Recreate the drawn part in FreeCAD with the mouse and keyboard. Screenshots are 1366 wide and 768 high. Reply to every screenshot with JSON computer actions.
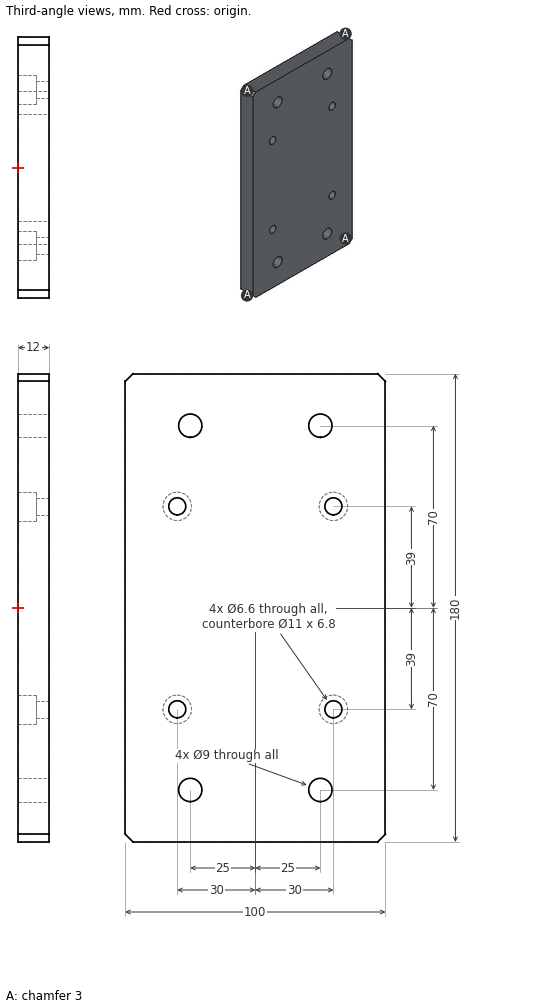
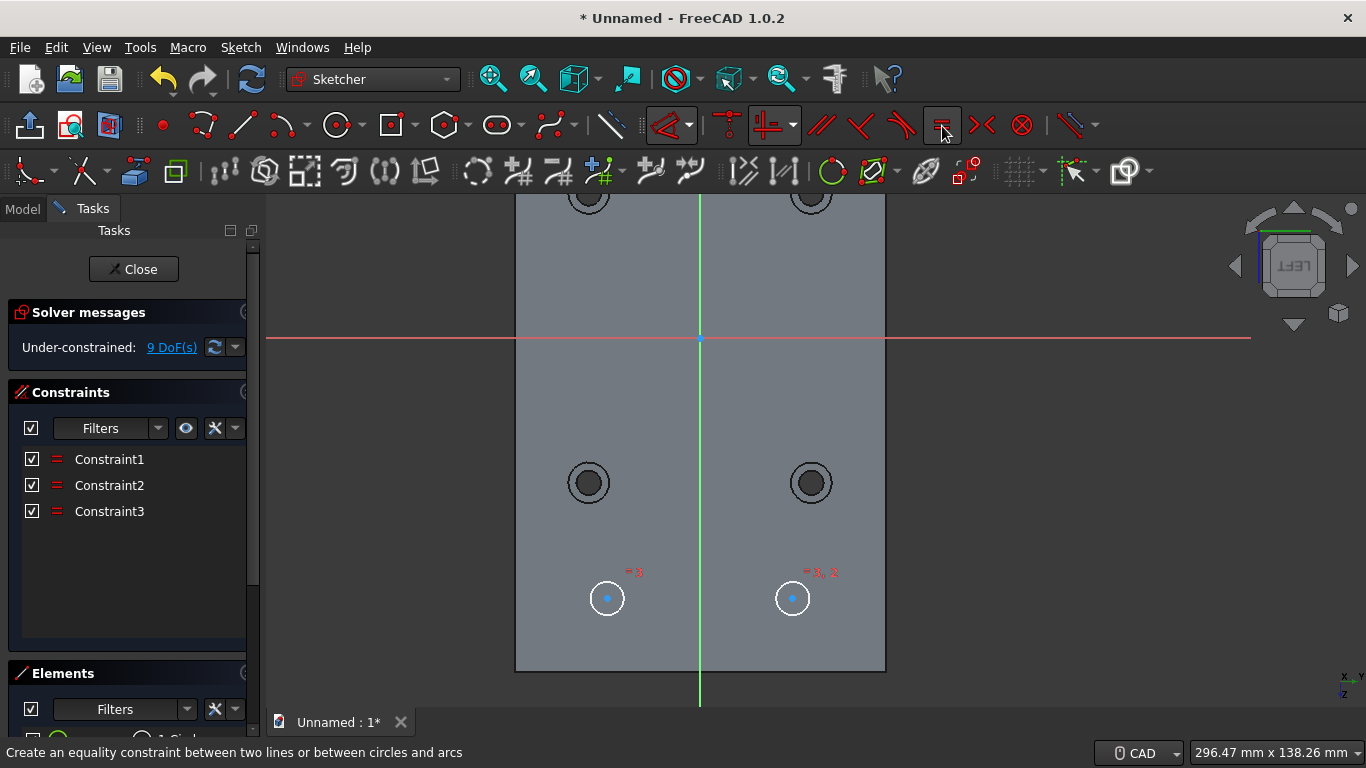
{"action": "scroll", "coordinate": [805, 587], "scroll_direction": "down", "scroll_amount": 3}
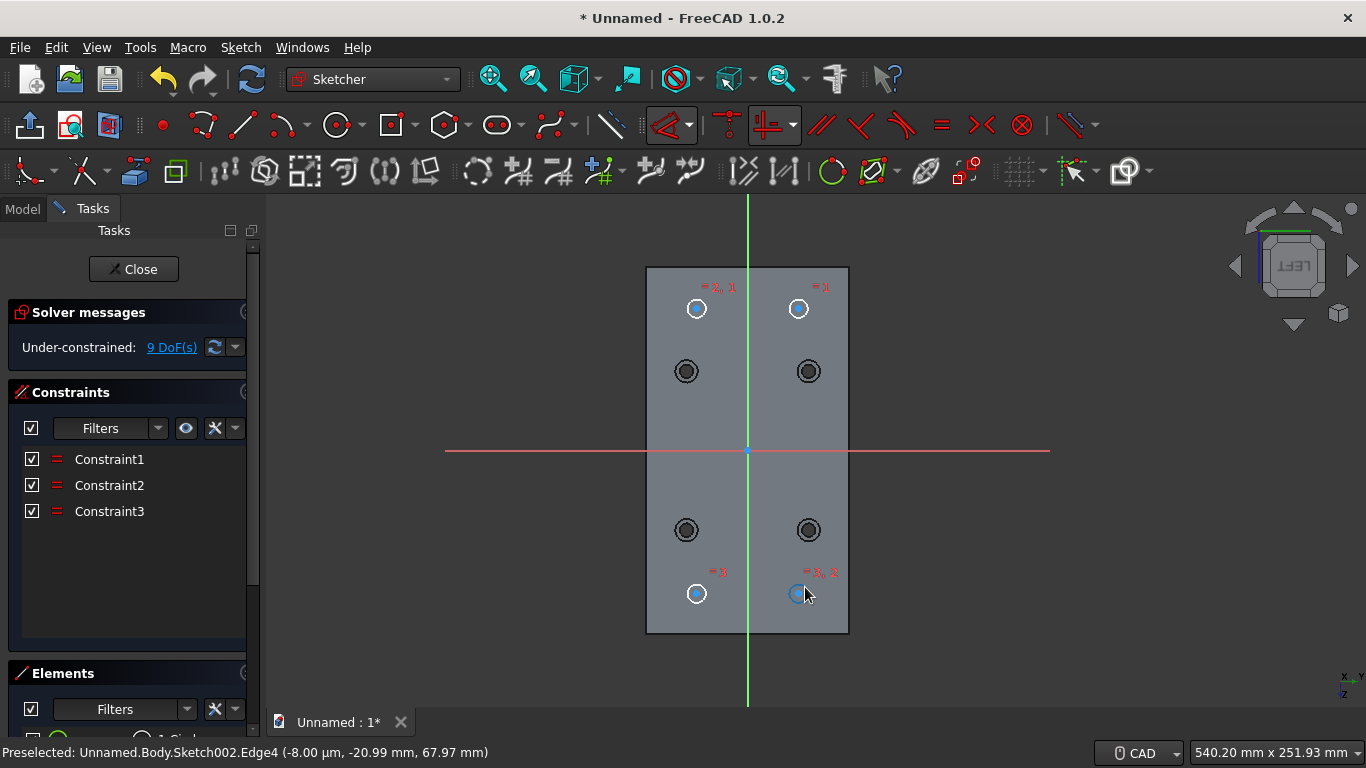
{"action": "left_click", "coordinate": [799, 309]}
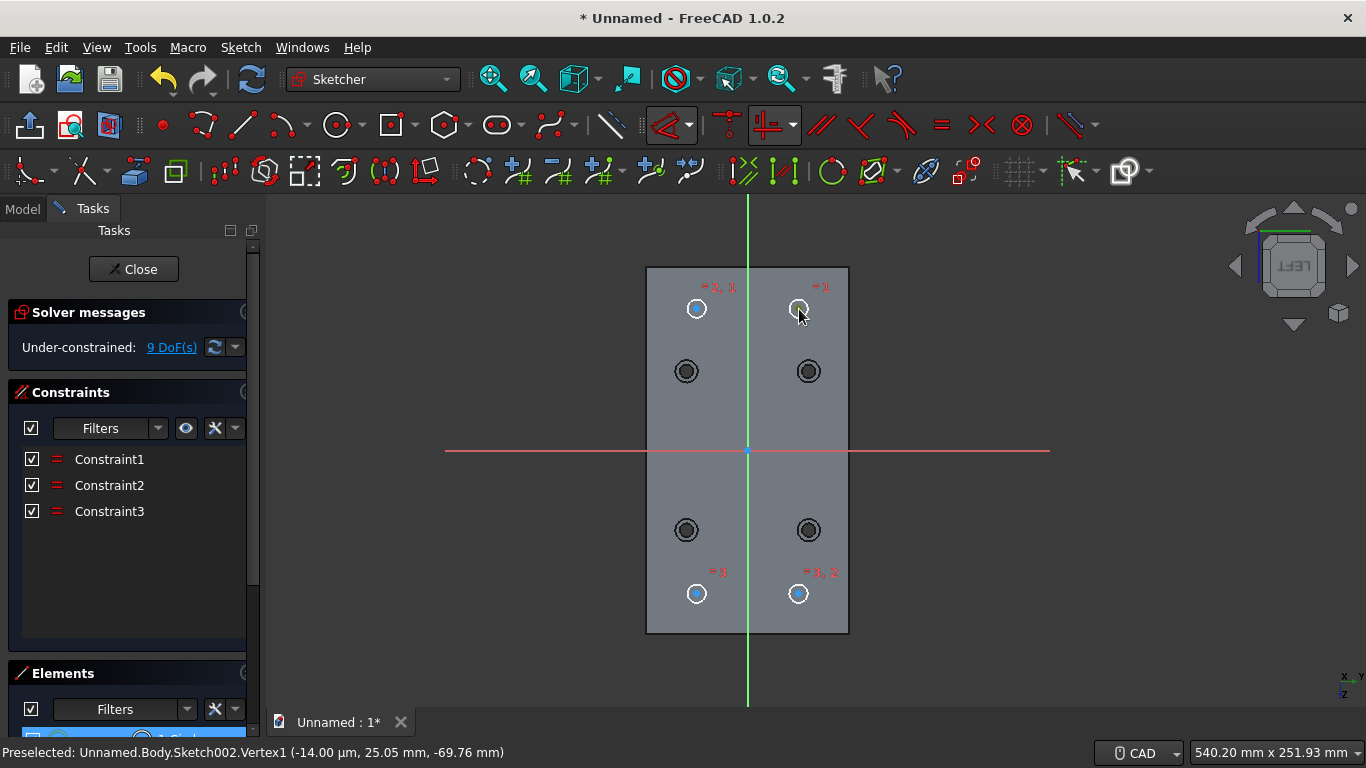
{"action": "left_click", "coordinate": [697, 309]}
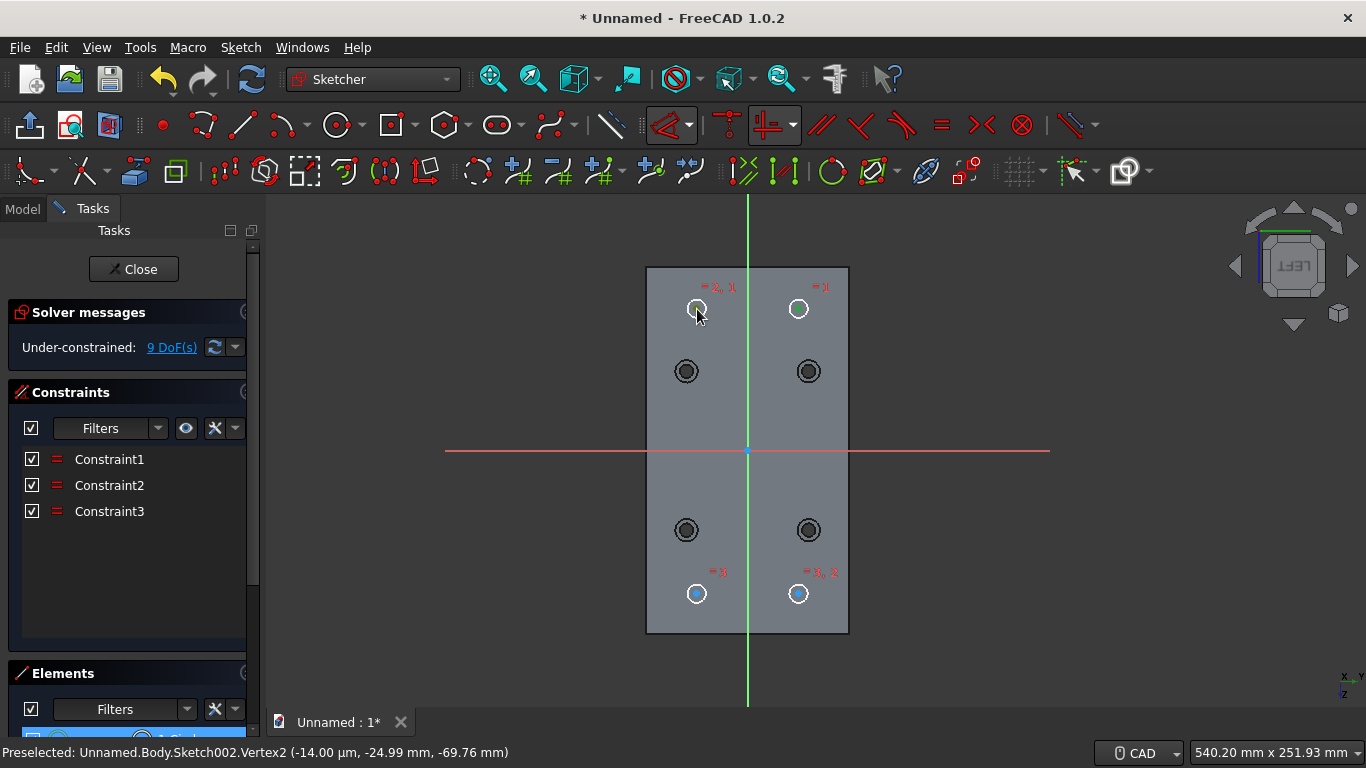
{"action": "left_click", "coordinate": [796, 126]}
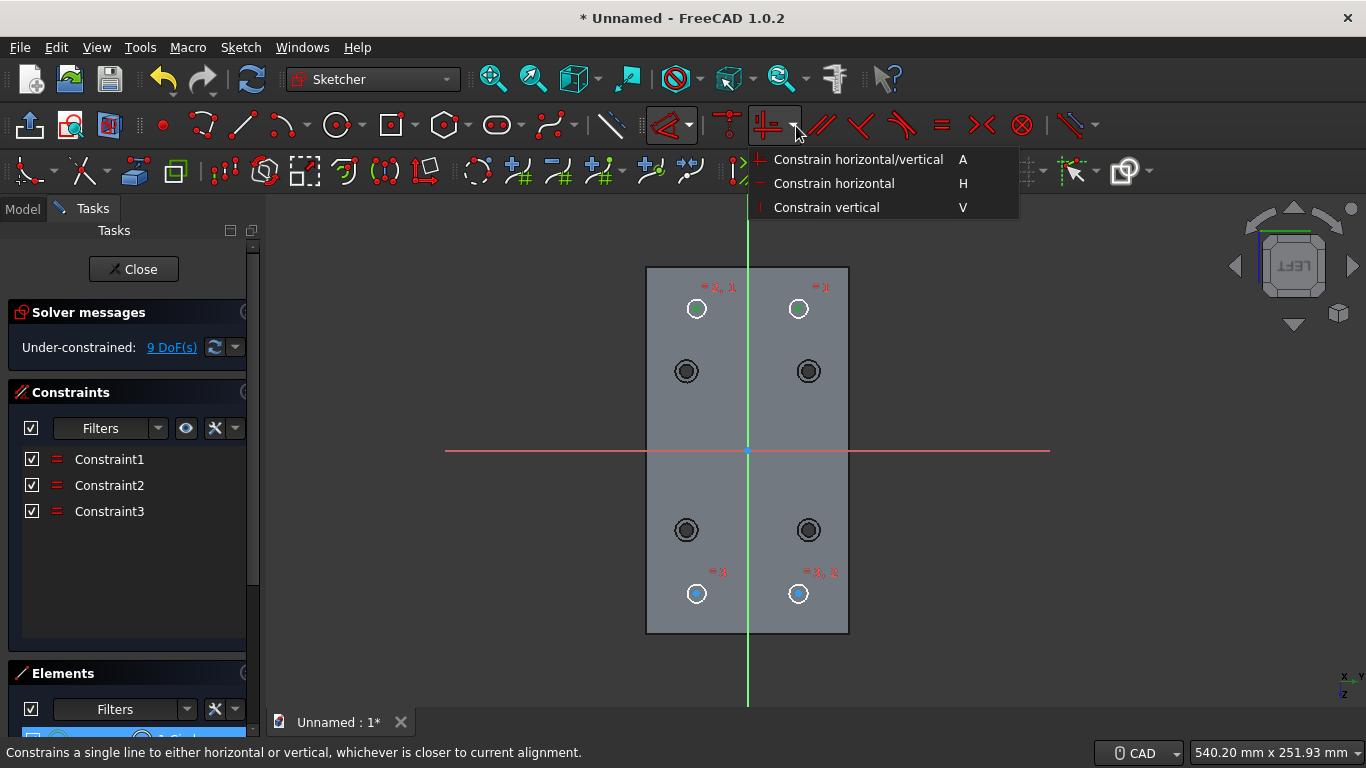
{"action": "left_click", "coordinate": [884, 183]}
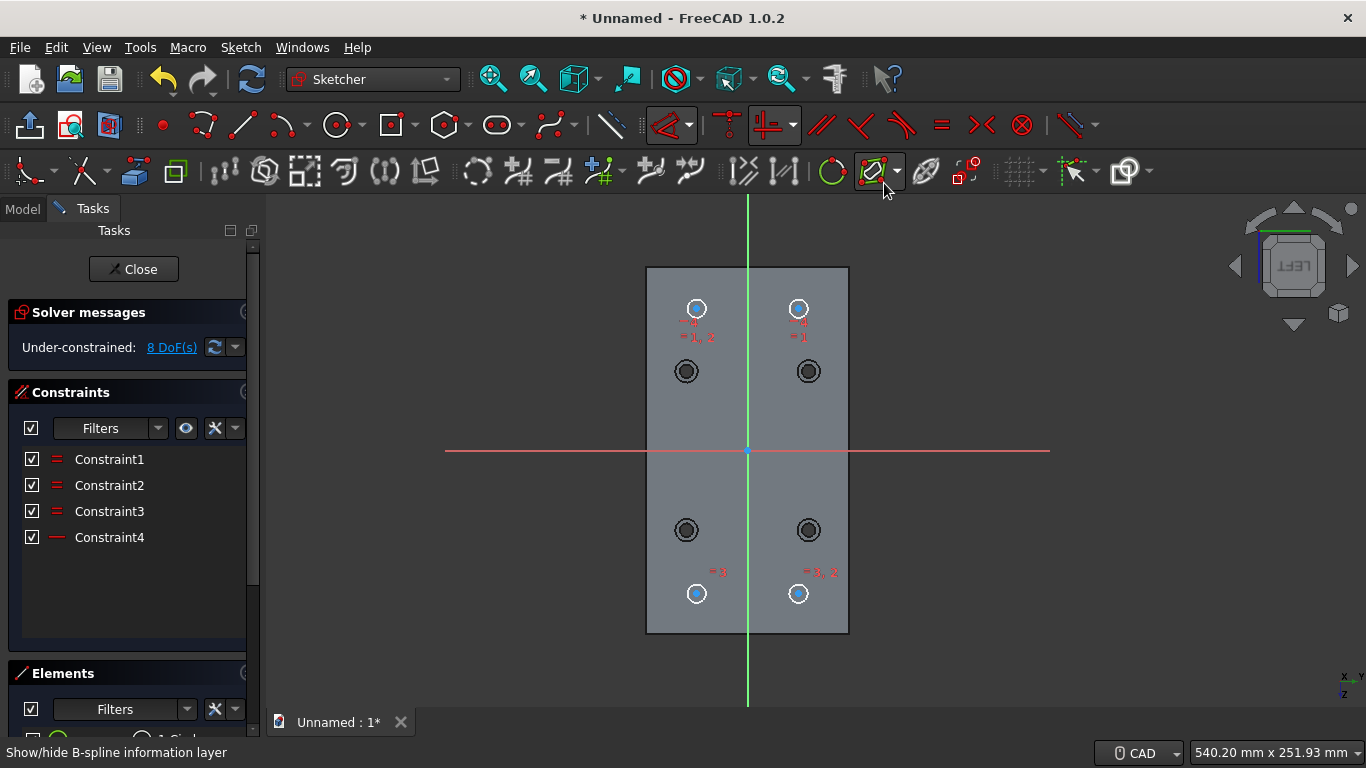
{"action": "left_click", "coordinate": [799, 309]}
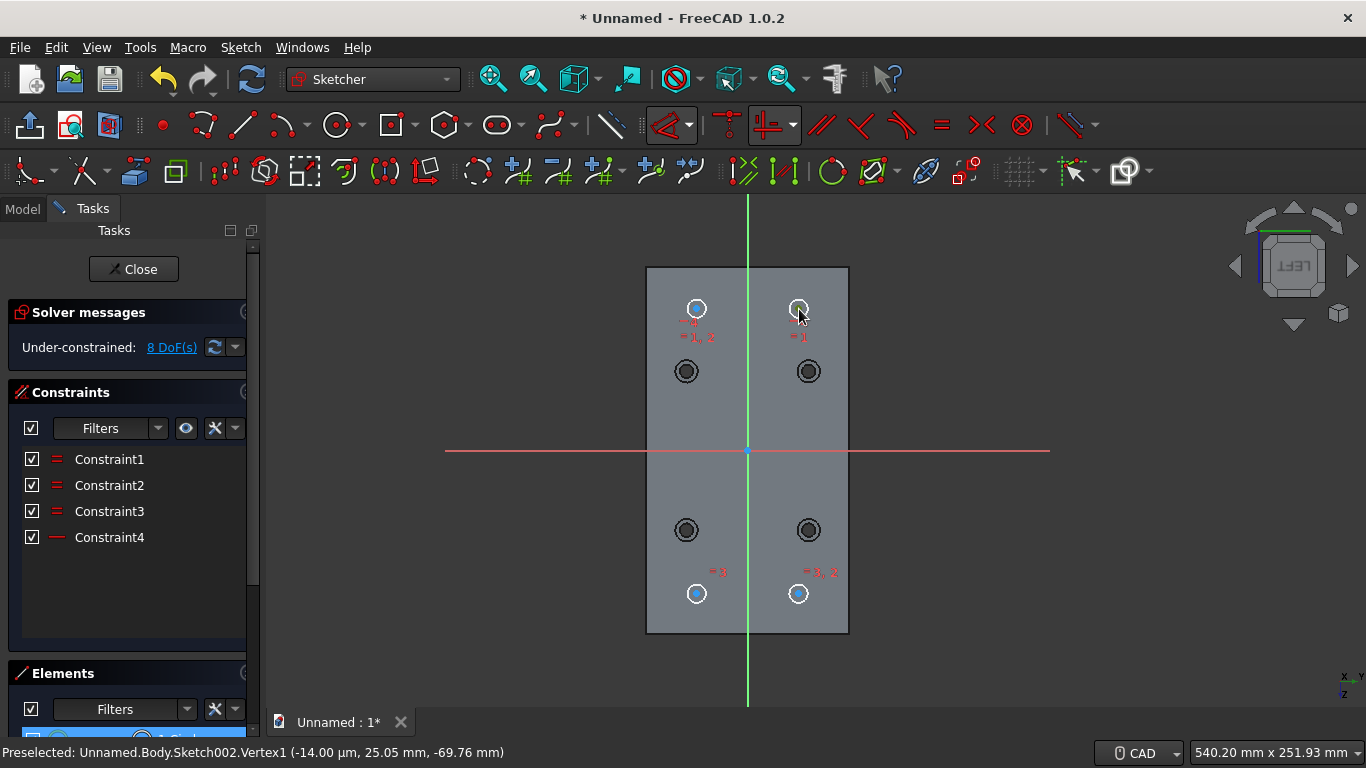
{"action": "left_click", "coordinate": [799, 594]}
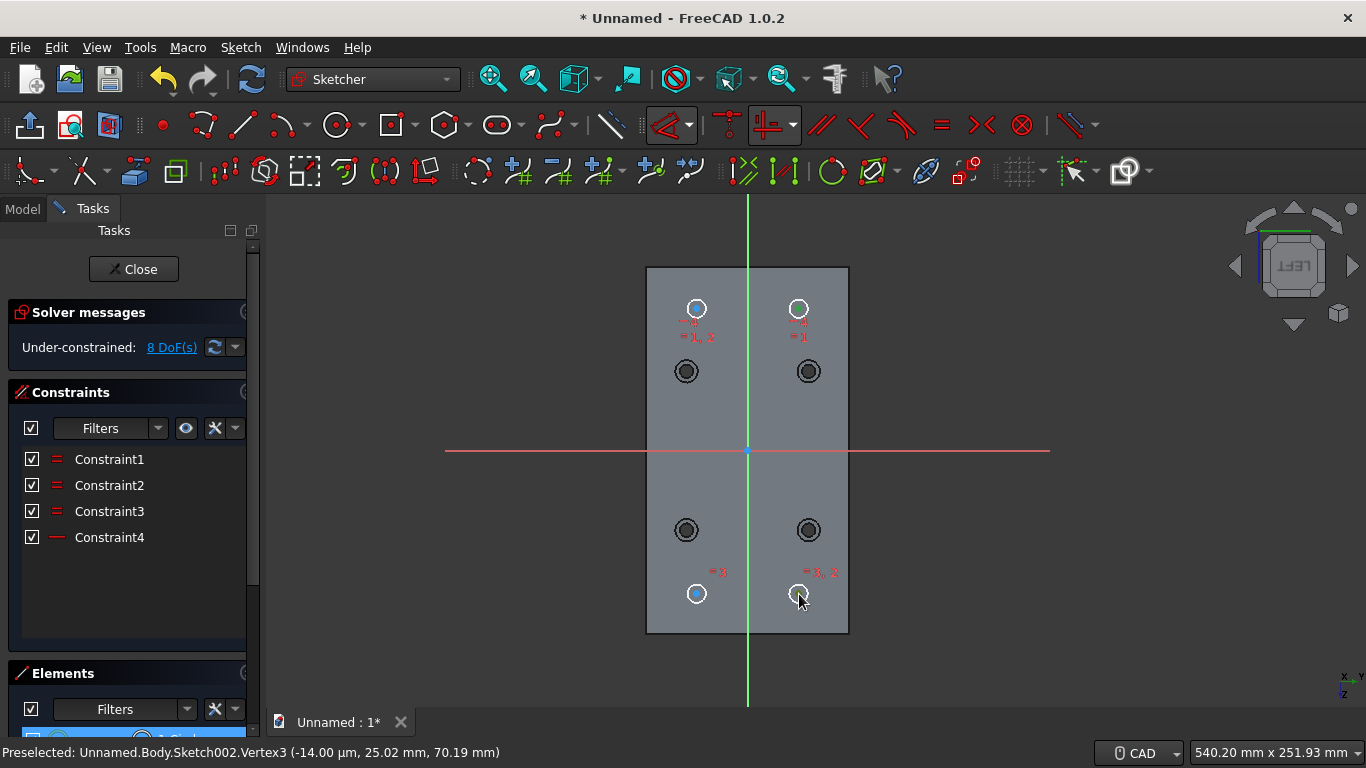
{"action": "key", "text": "v"}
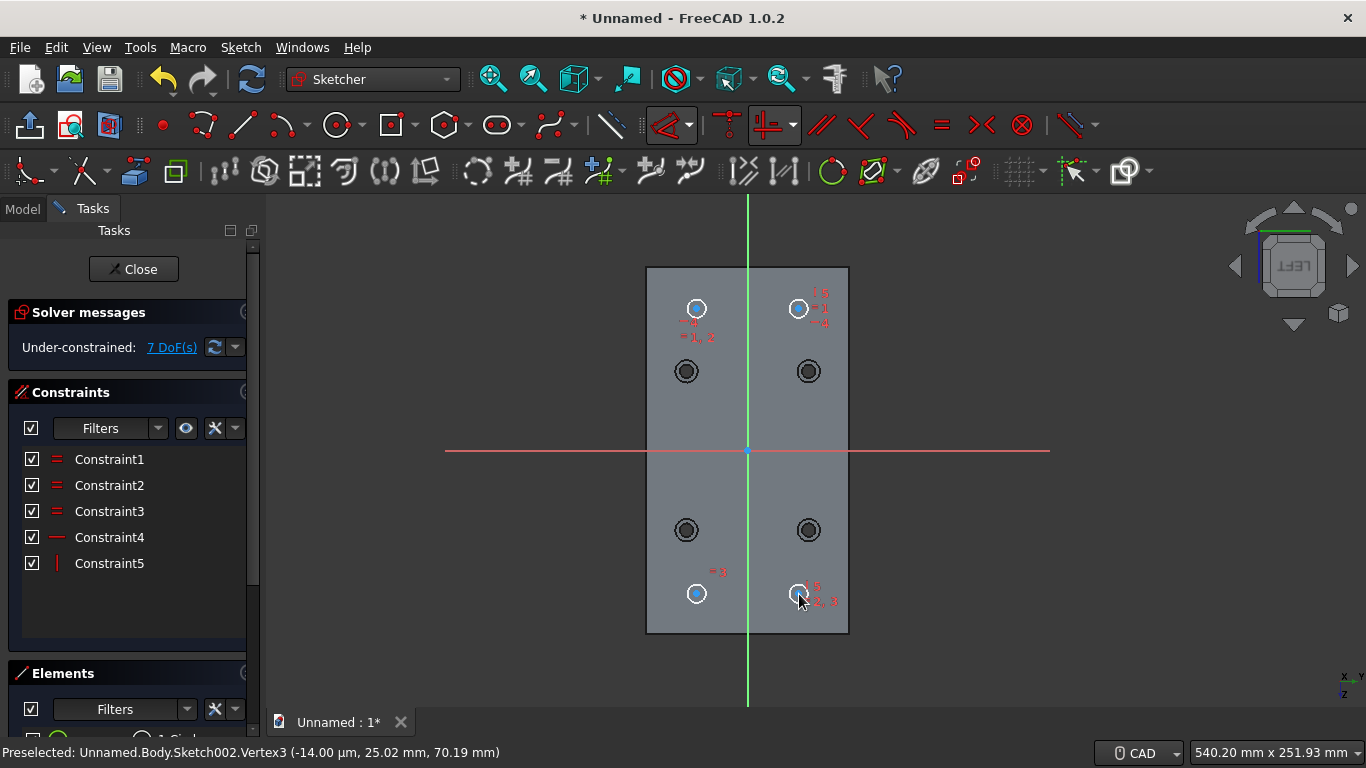
{"action": "left_click", "coordinate": [697, 309]}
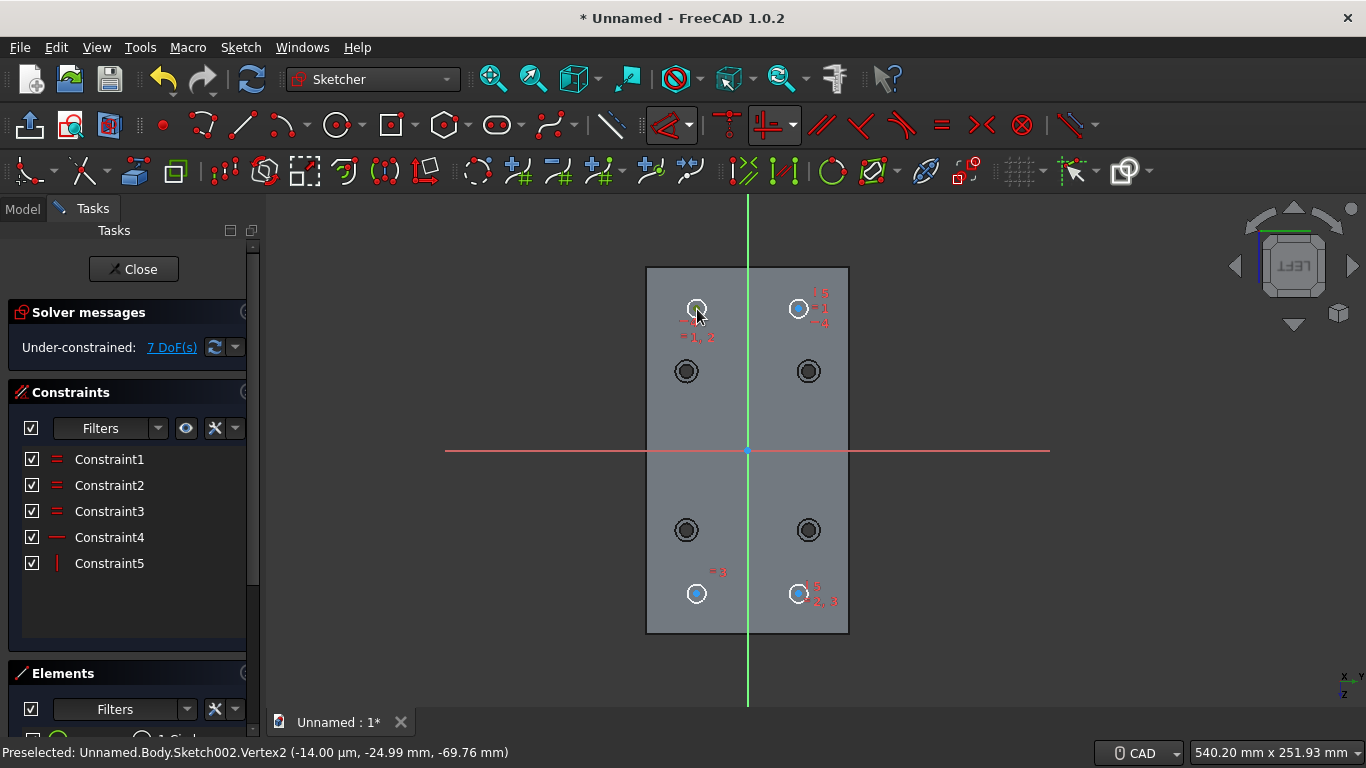
{"action": "left_click", "coordinate": [697, 594]}